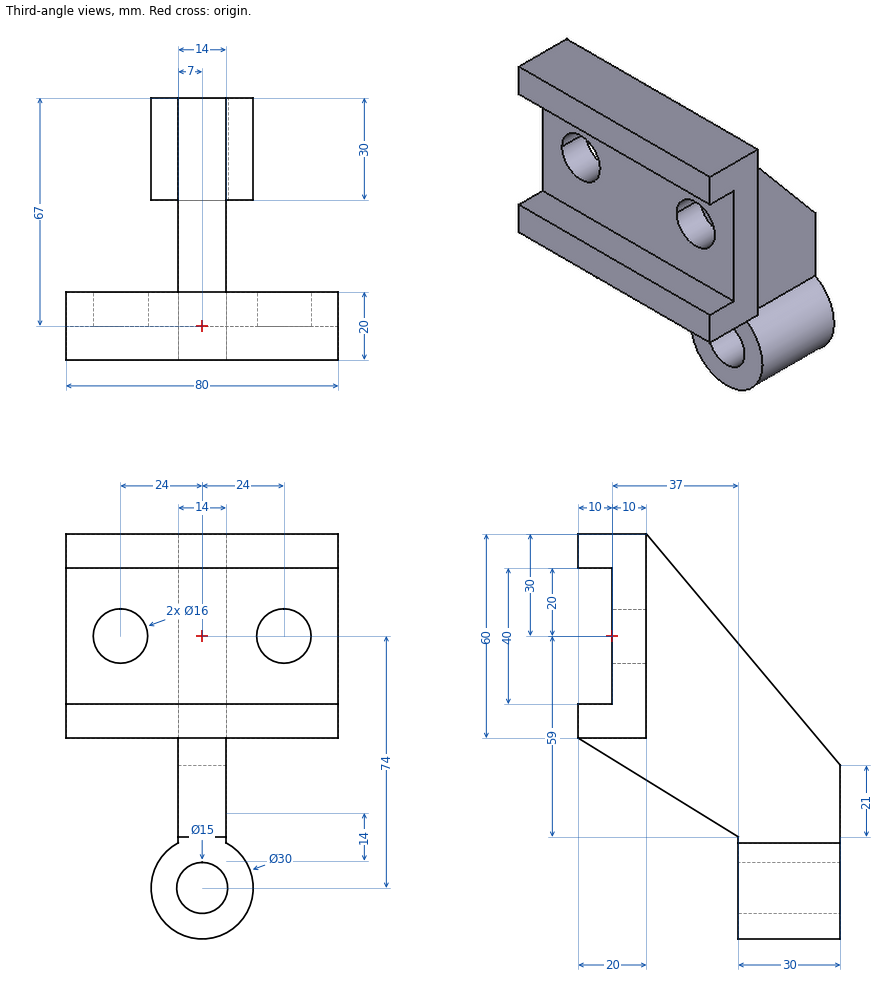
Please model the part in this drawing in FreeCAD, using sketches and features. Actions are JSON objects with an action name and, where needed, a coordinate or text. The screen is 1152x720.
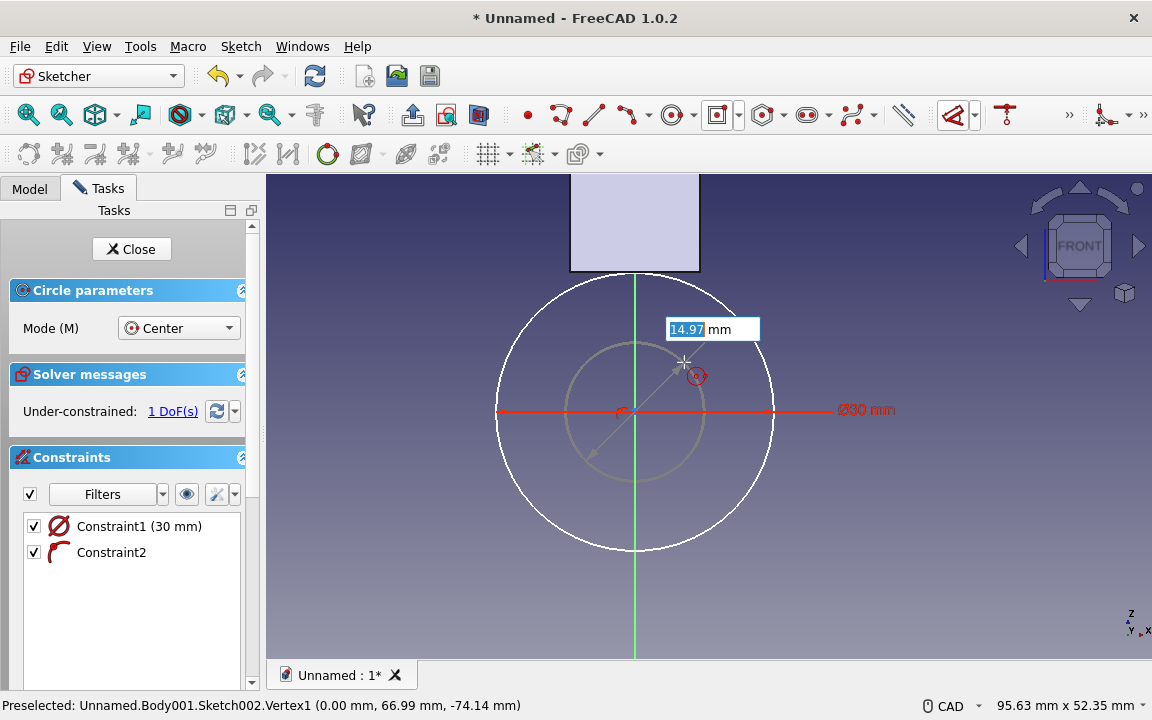
{"action": "type", "text": "15"}
{"action": "key", "text": "Return"}
{"action": "key", "text": "Escape"}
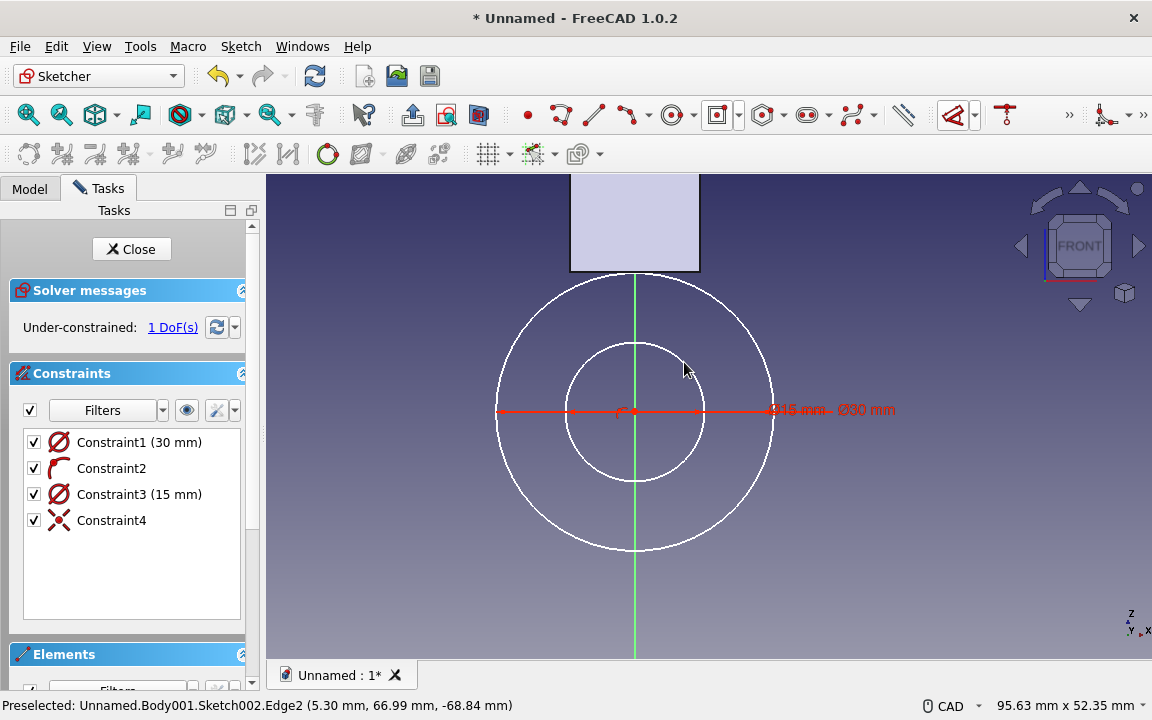
{"action": "left_click", "coordinate": [635, 412]}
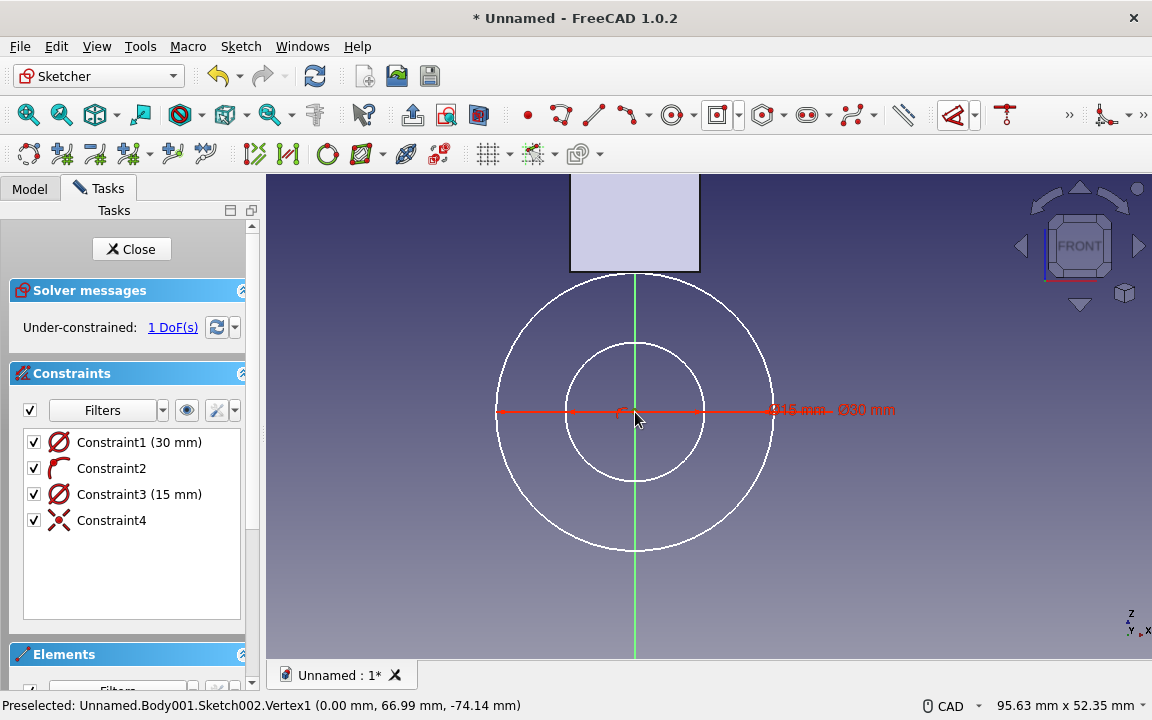
{"action": "left_click", "coordinate": [974, 116]}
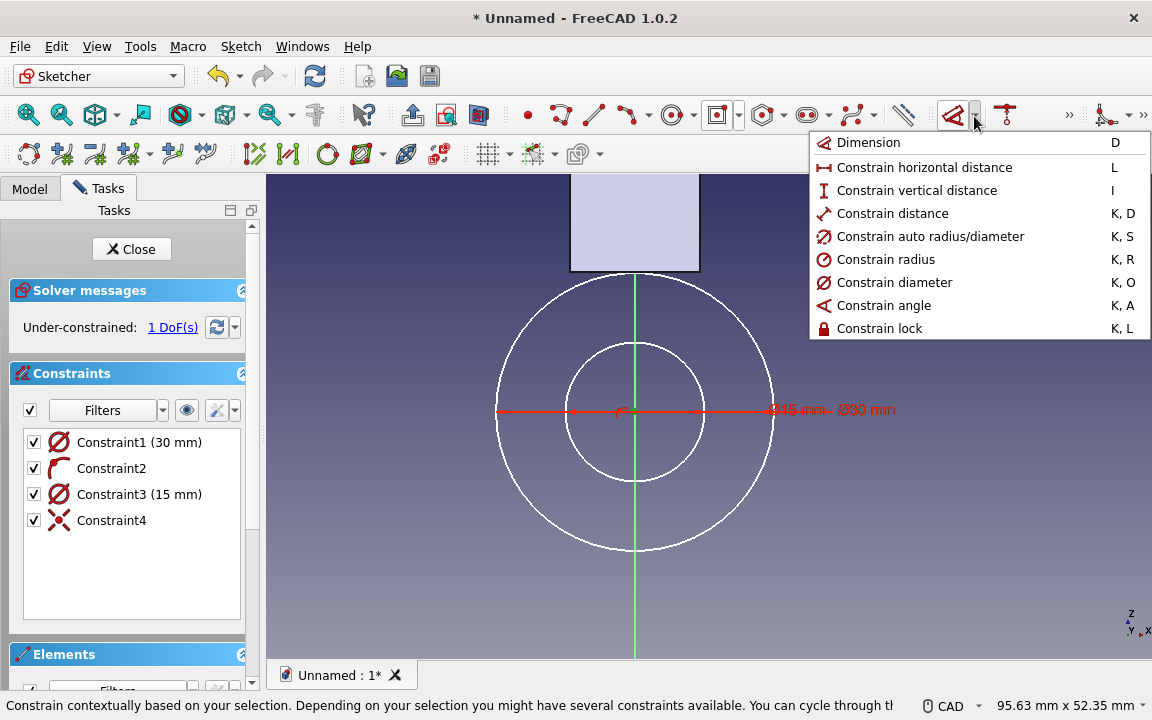
{"action": "left_click", "coordinate": [980, 190]}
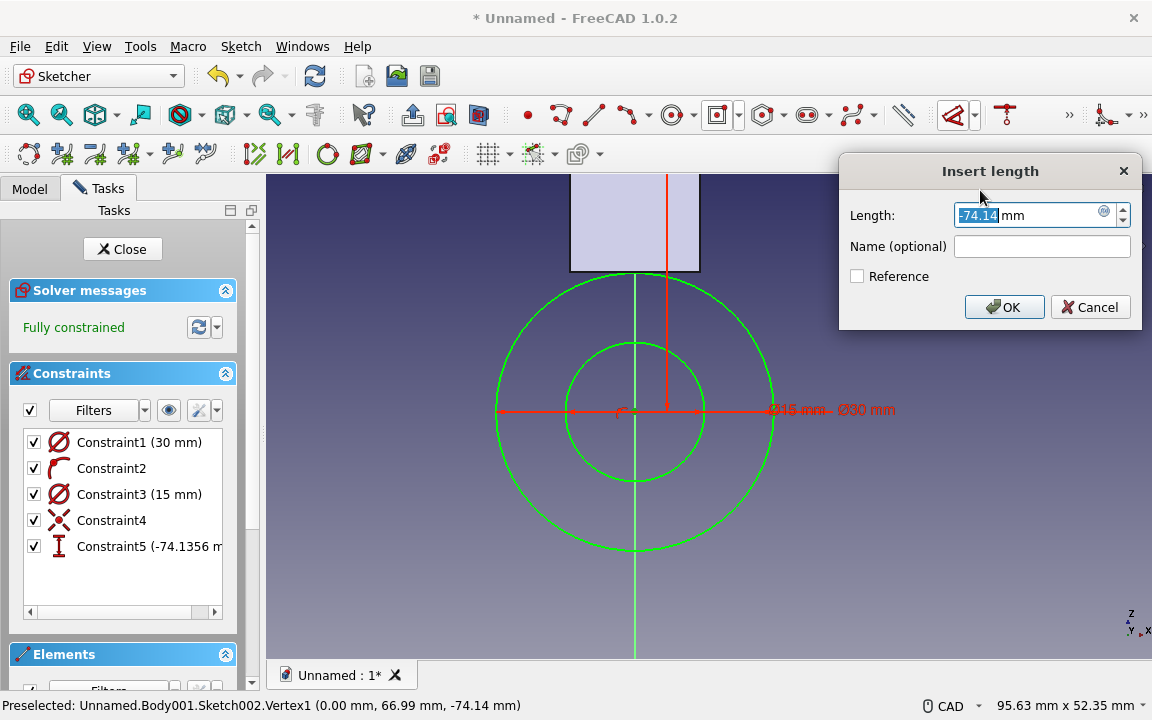
{"action": "type", "text": "-74"}
{"action": "key", "text": "Return"}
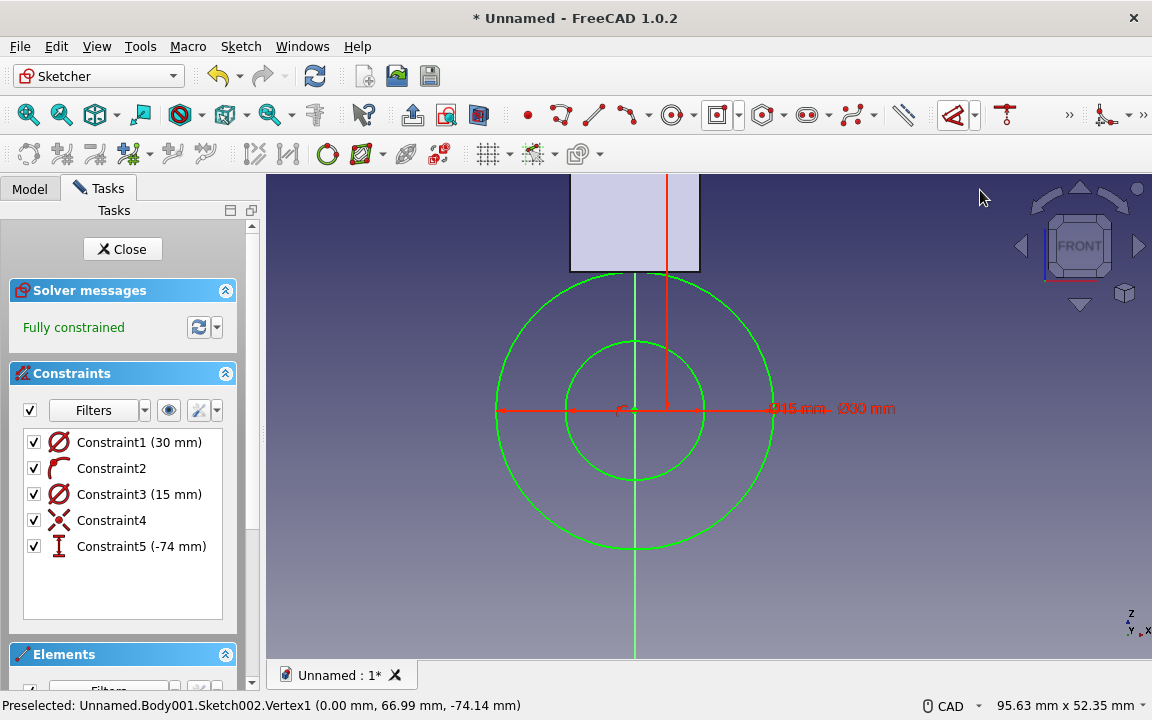
{"action": "left_click", "coordinate": [123, 249]}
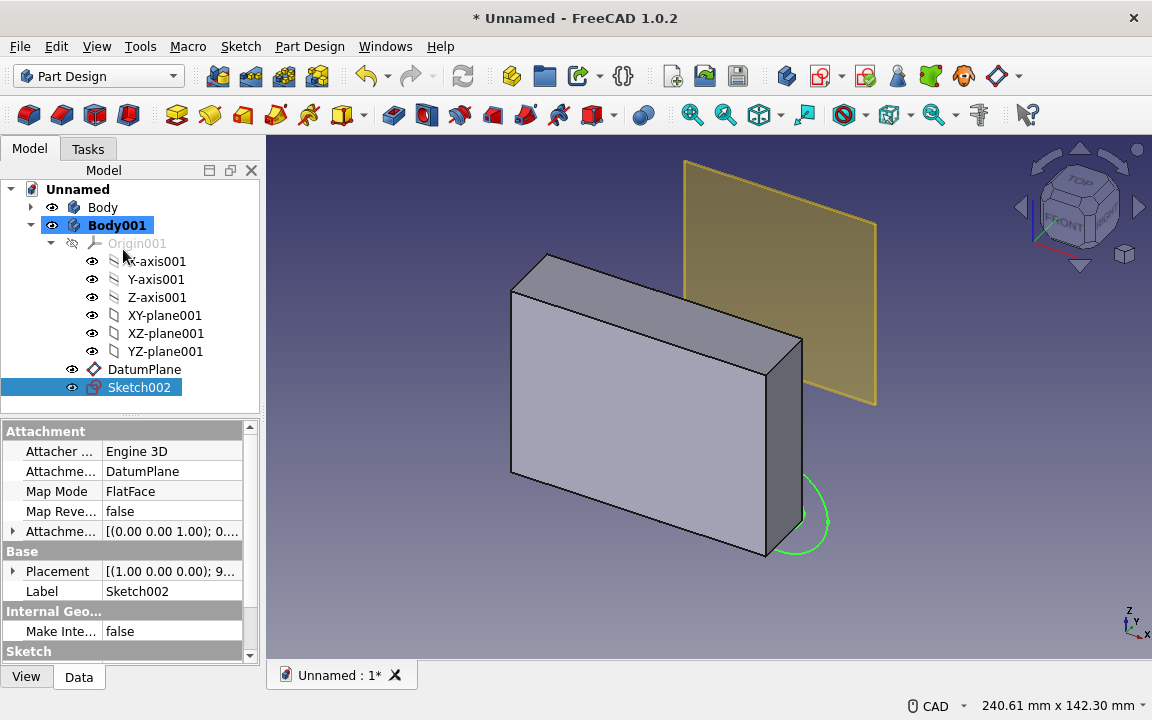
{"action": "left_click", "coordinate": [177, 116]}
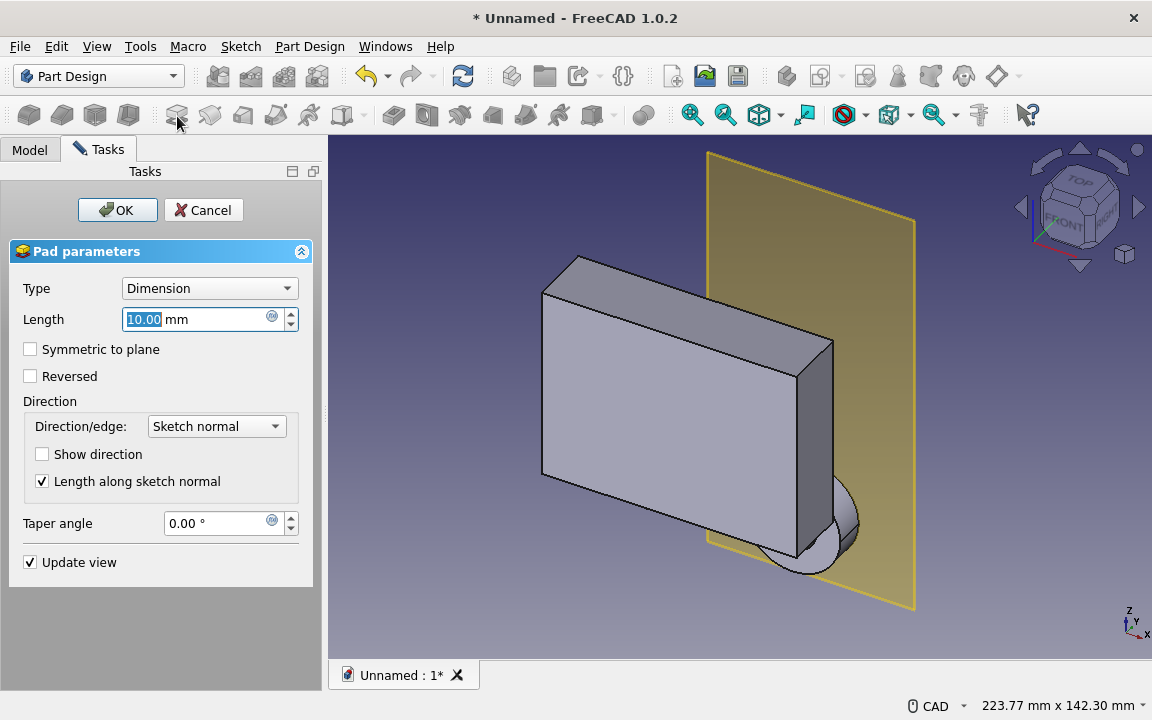
{"action": "type", "text": "30"}
{"action": "key", "text": "Tab"}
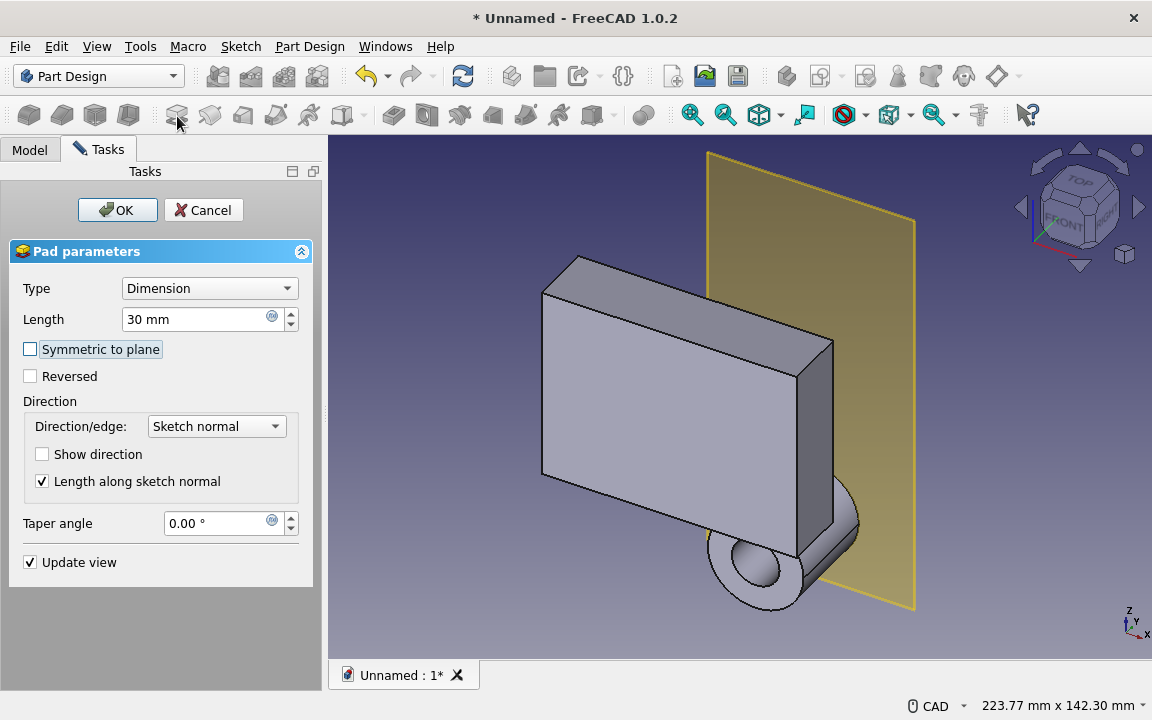
{"action": "left_click", "coordinate": [118, 210]}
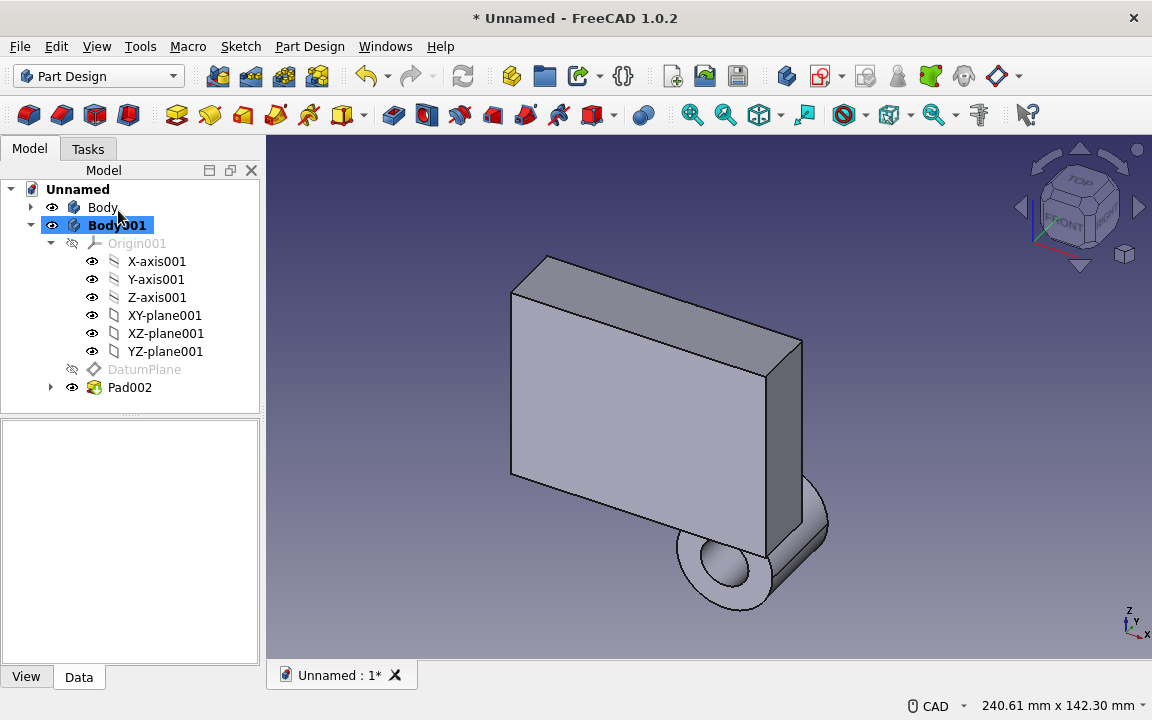
{"action": "left_click", "coordinate": [693, 116]}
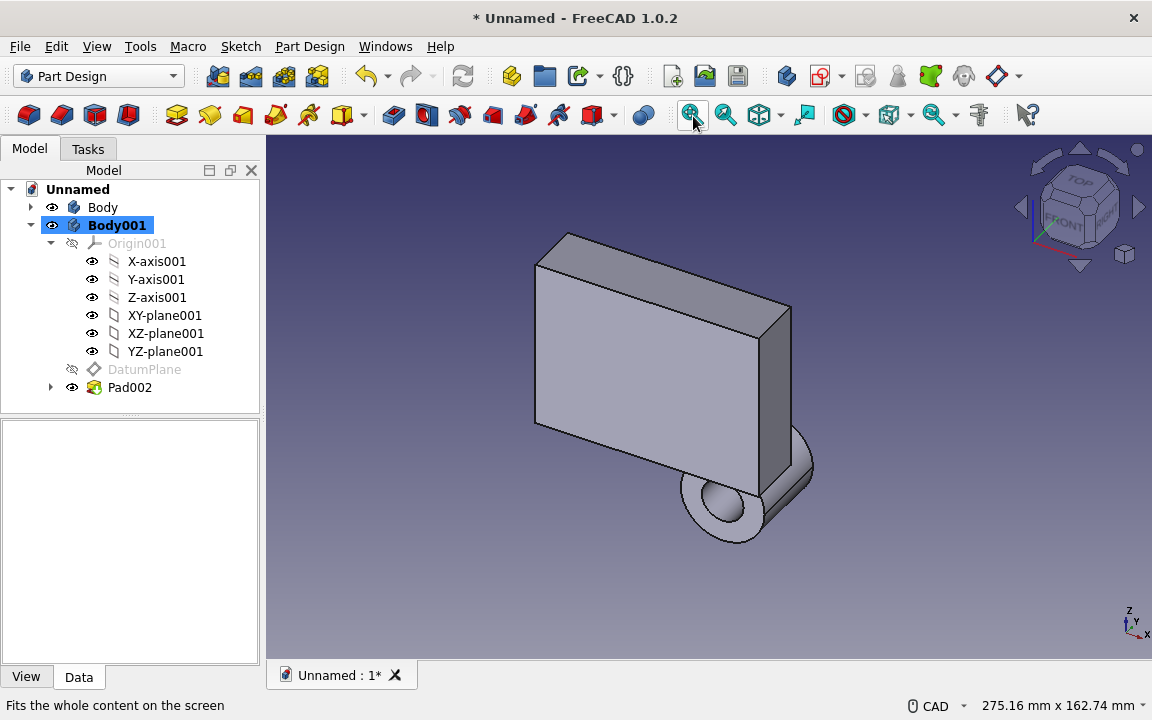
{"action": "double_click", "coordinate": [97, 207]}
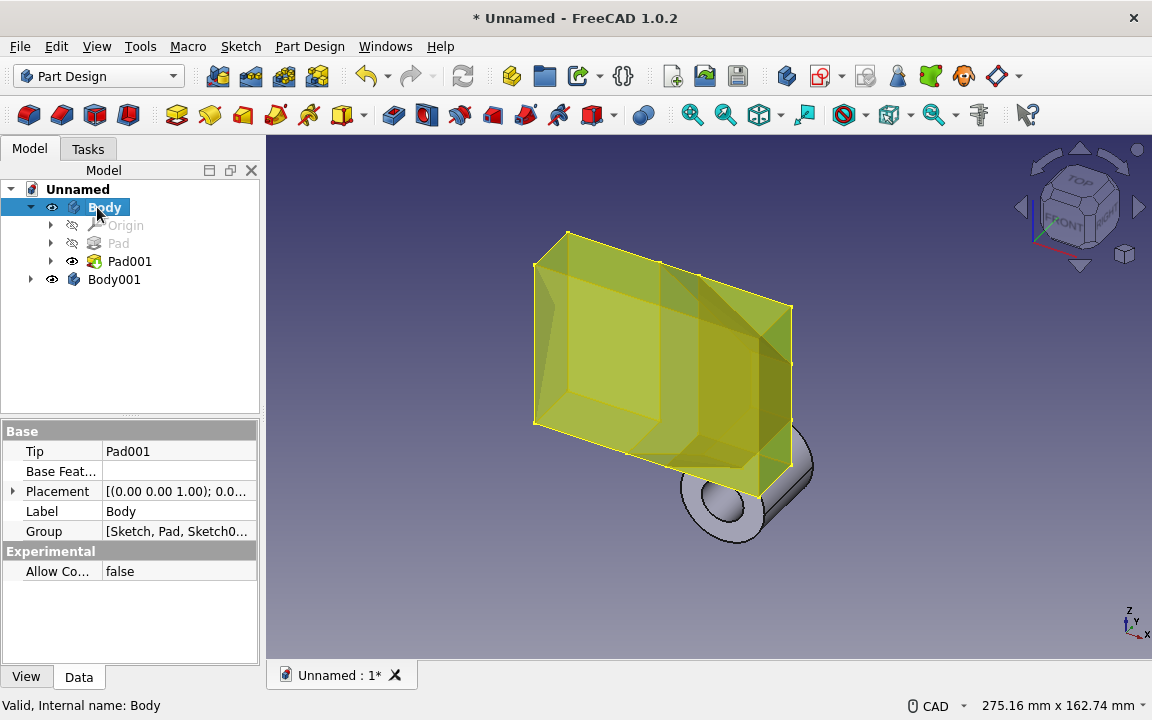
{"action": "left_click", "coordinate": [97, 207]}